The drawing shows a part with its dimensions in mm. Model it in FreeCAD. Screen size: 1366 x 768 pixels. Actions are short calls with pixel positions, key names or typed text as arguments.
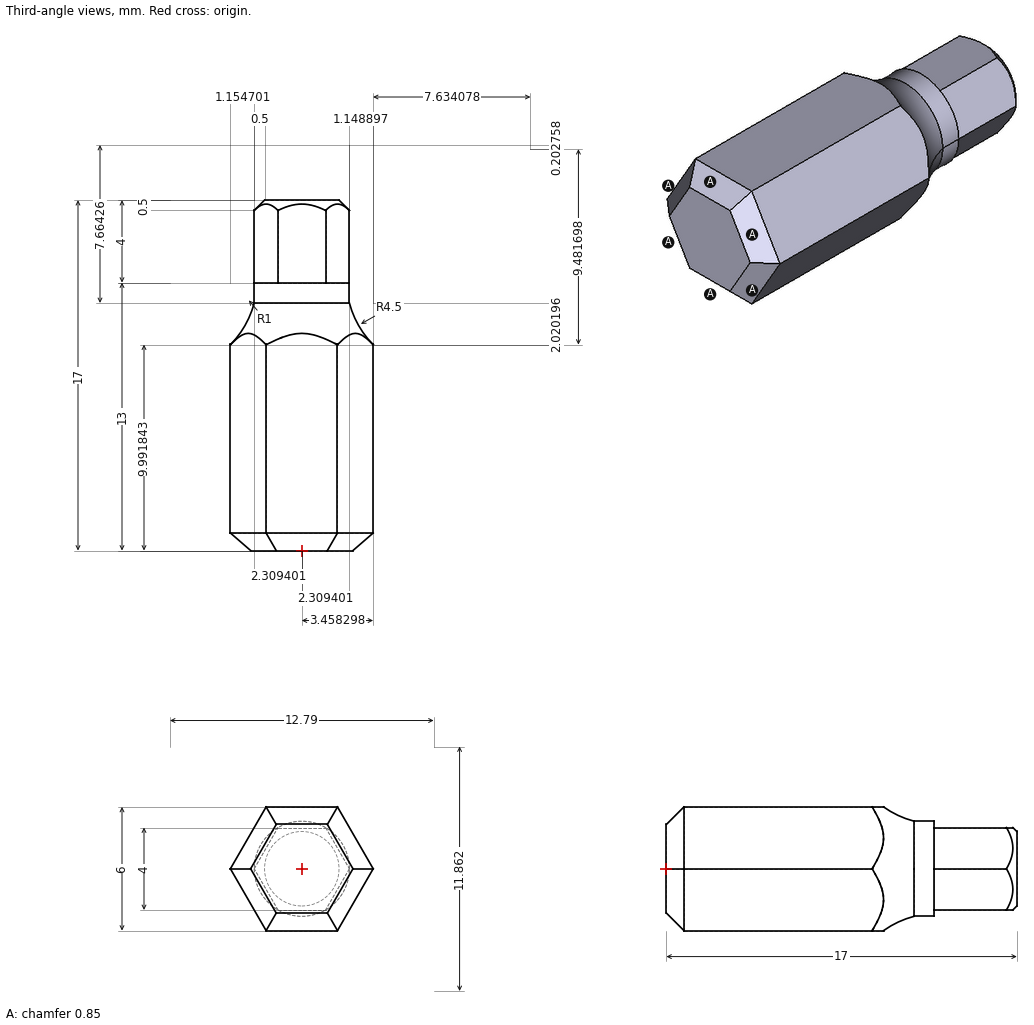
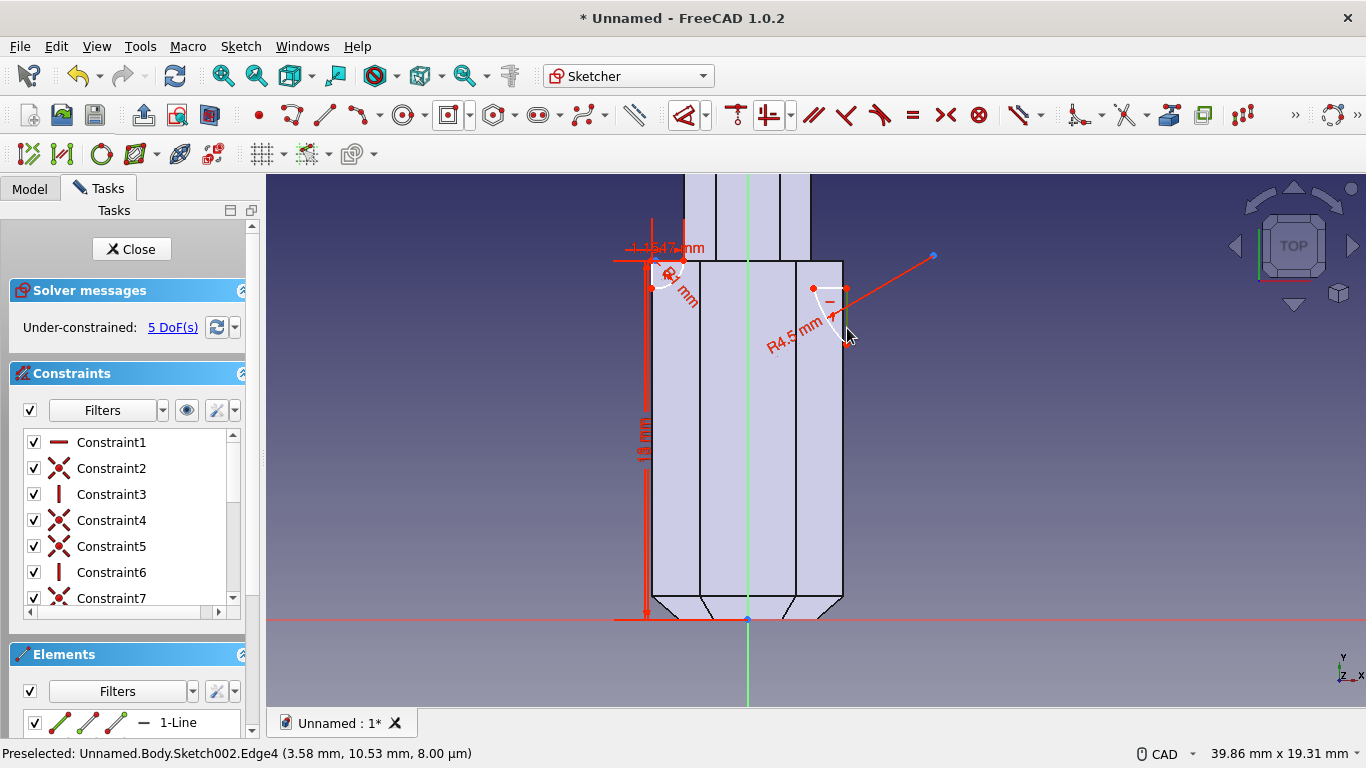
click(706, 116)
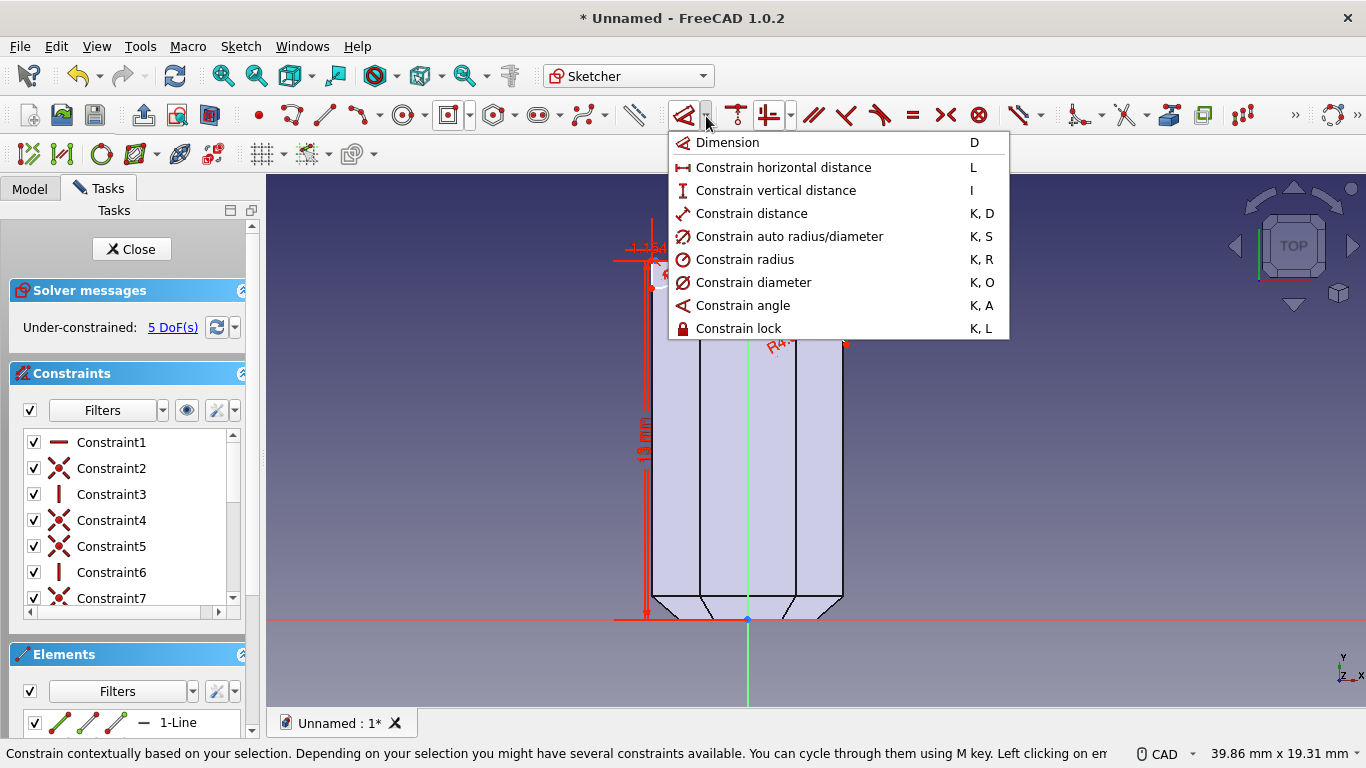
click(839, 190)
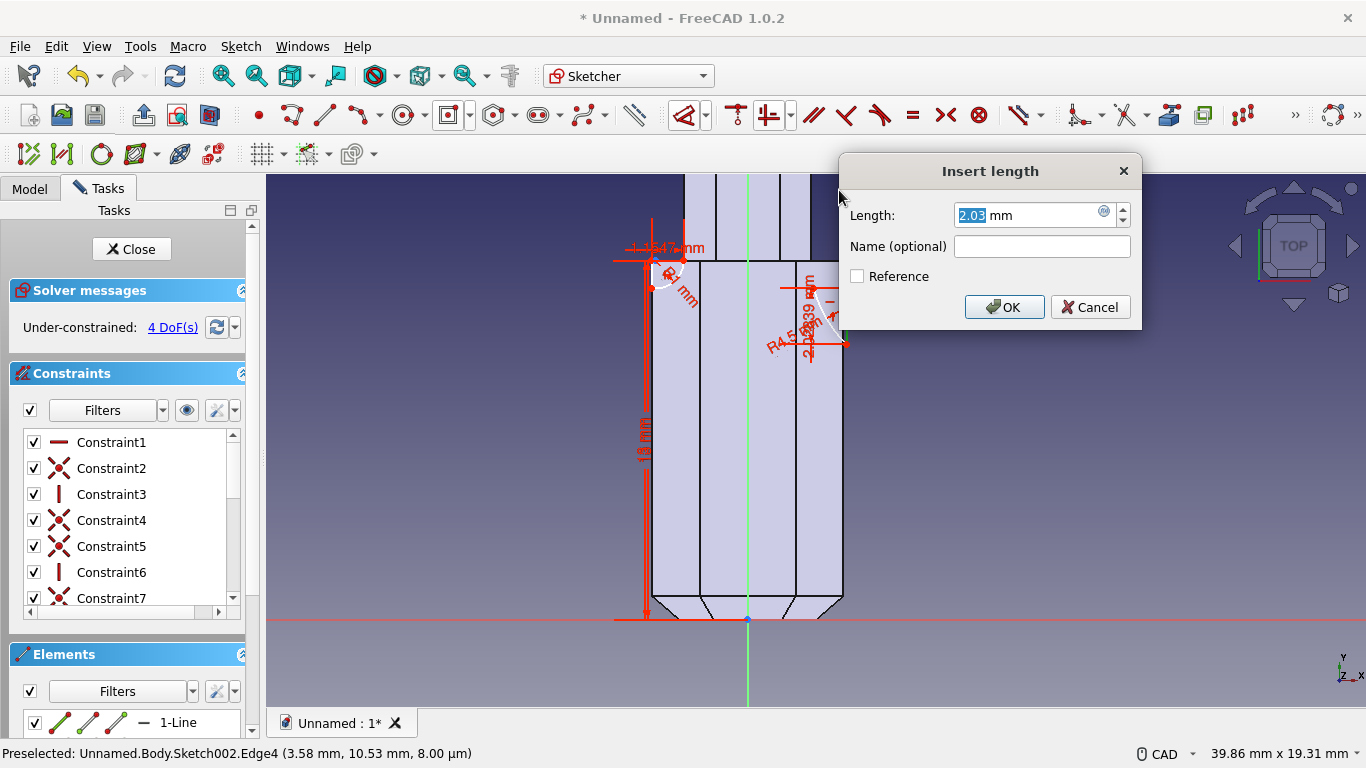
text(2.020196)
key(Return)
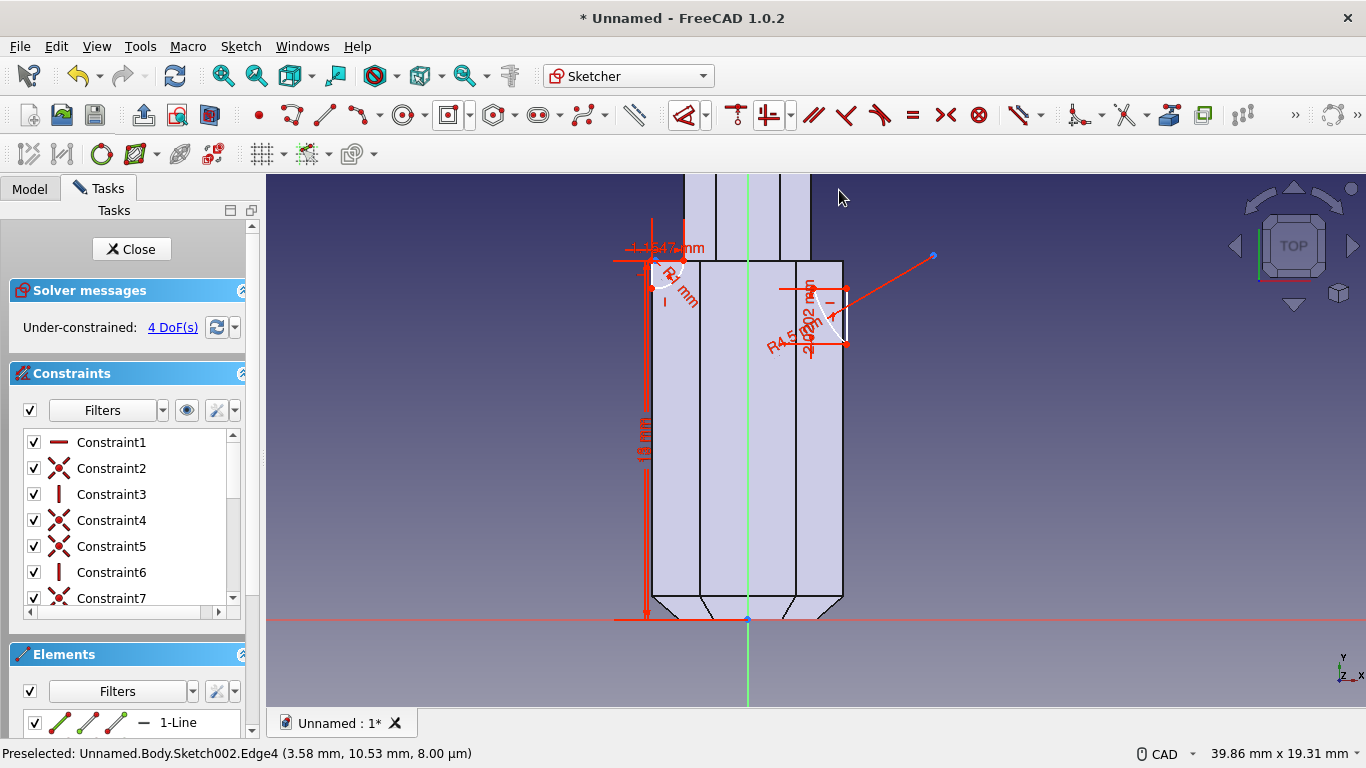
scroll(837, 289, up, 2)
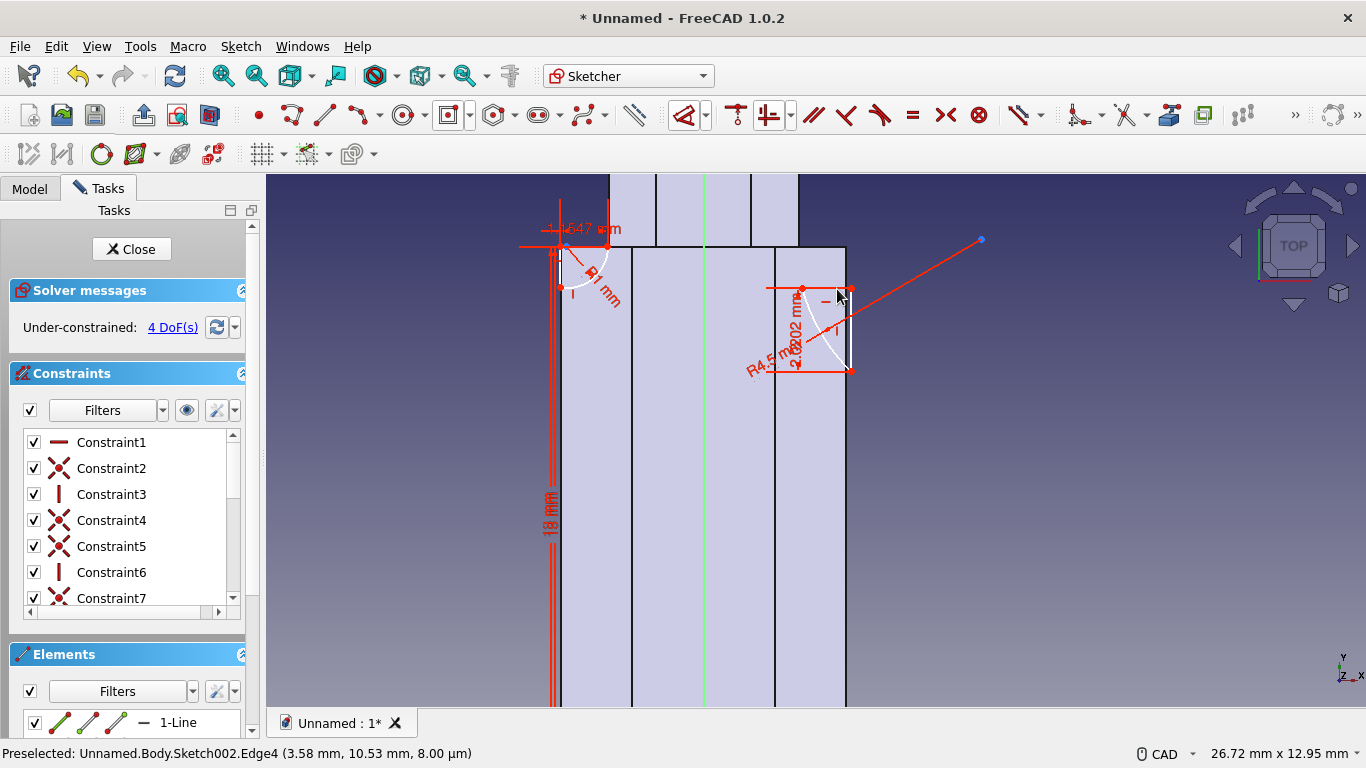
click(836, 288)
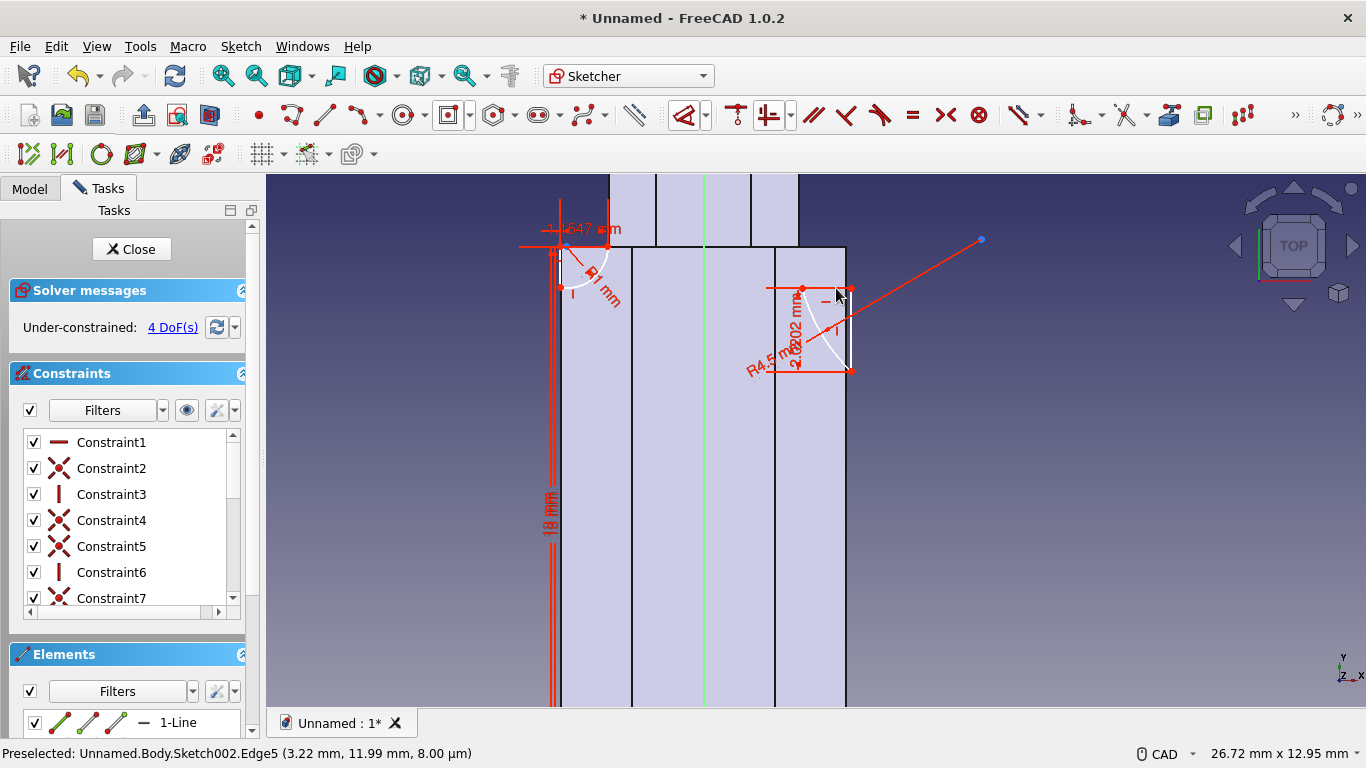
click(706, 116)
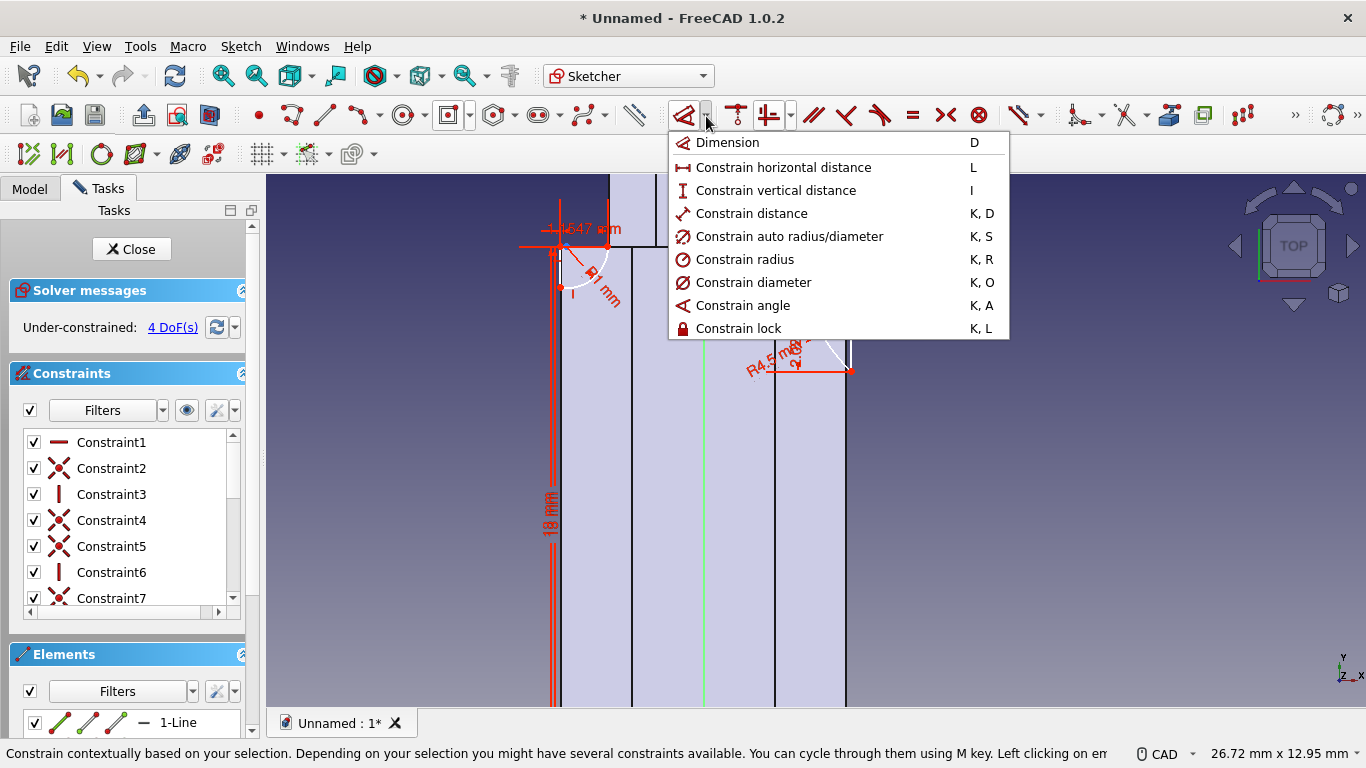
click(839, 168)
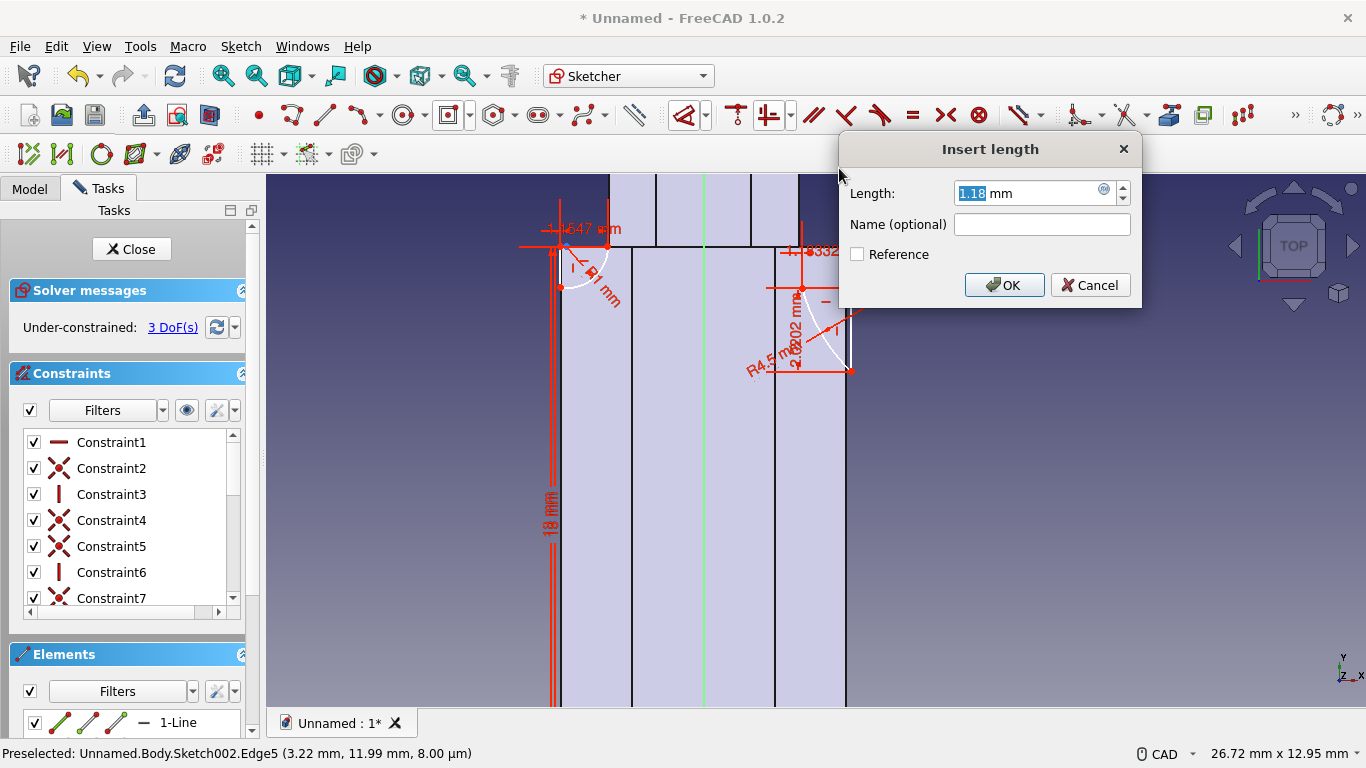
text(1.148897)
key(Return)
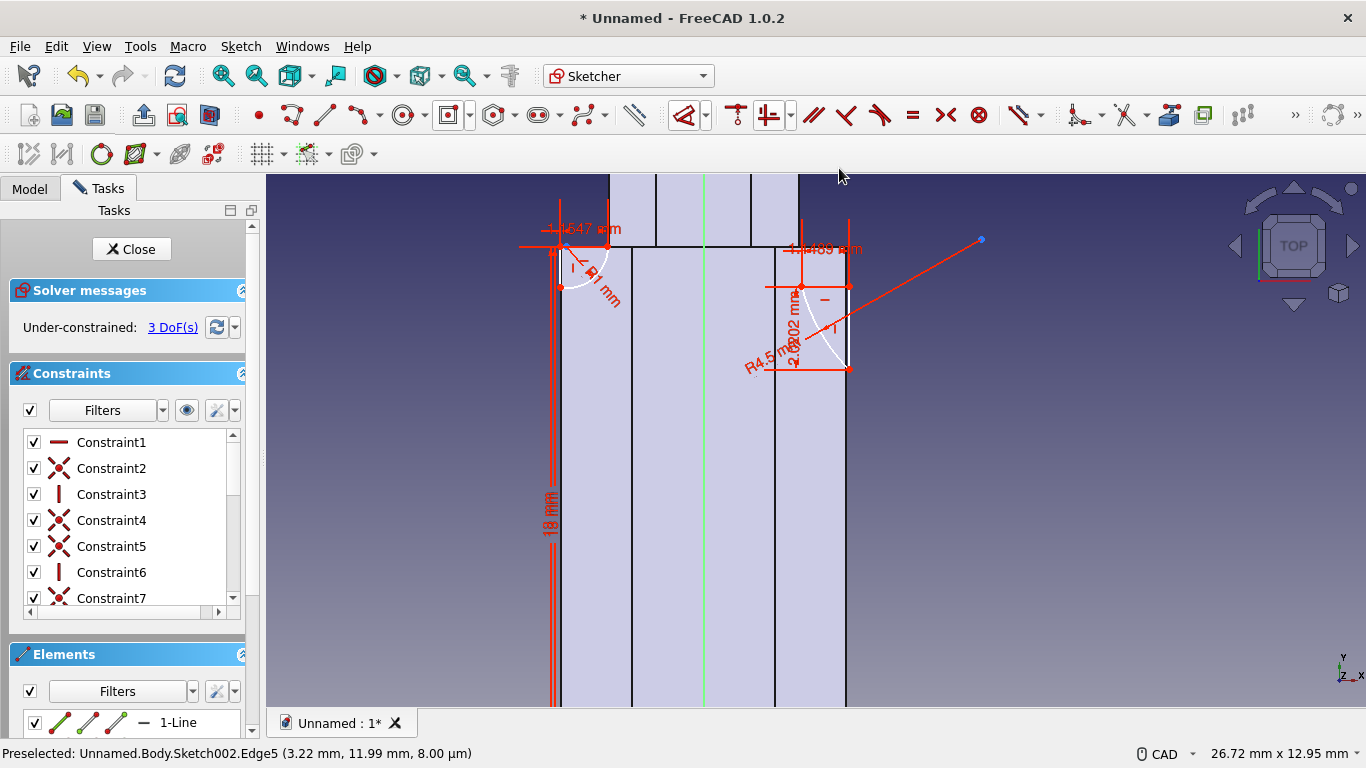
click(608, 247)